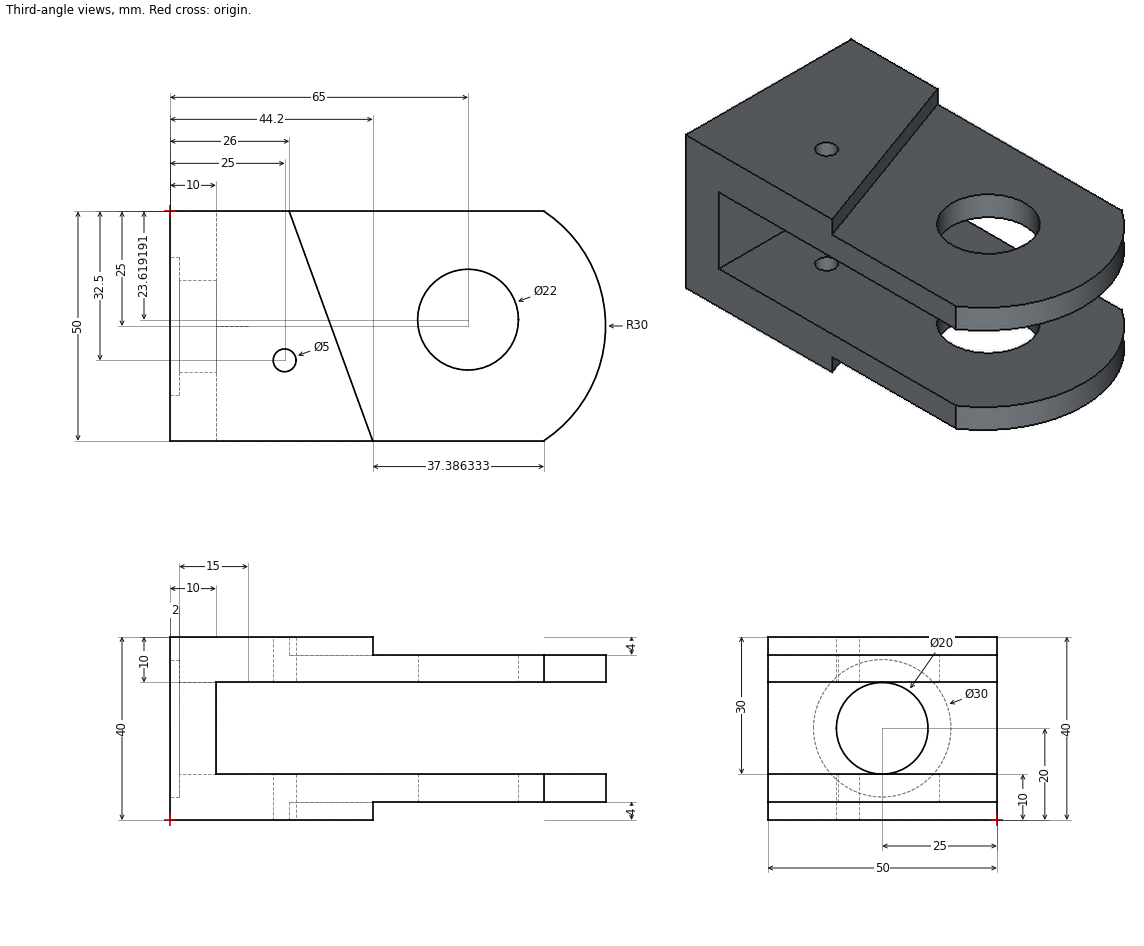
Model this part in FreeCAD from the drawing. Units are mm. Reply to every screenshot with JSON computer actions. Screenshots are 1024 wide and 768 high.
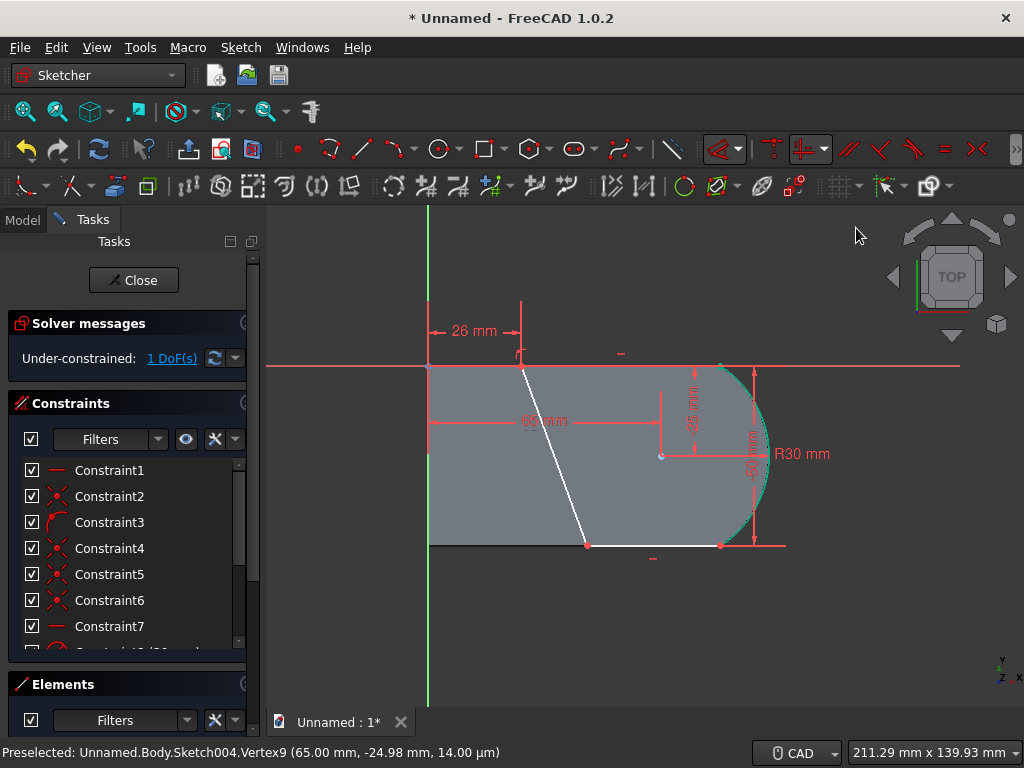
{"action": "left_click", "coordinate": [587, 546]}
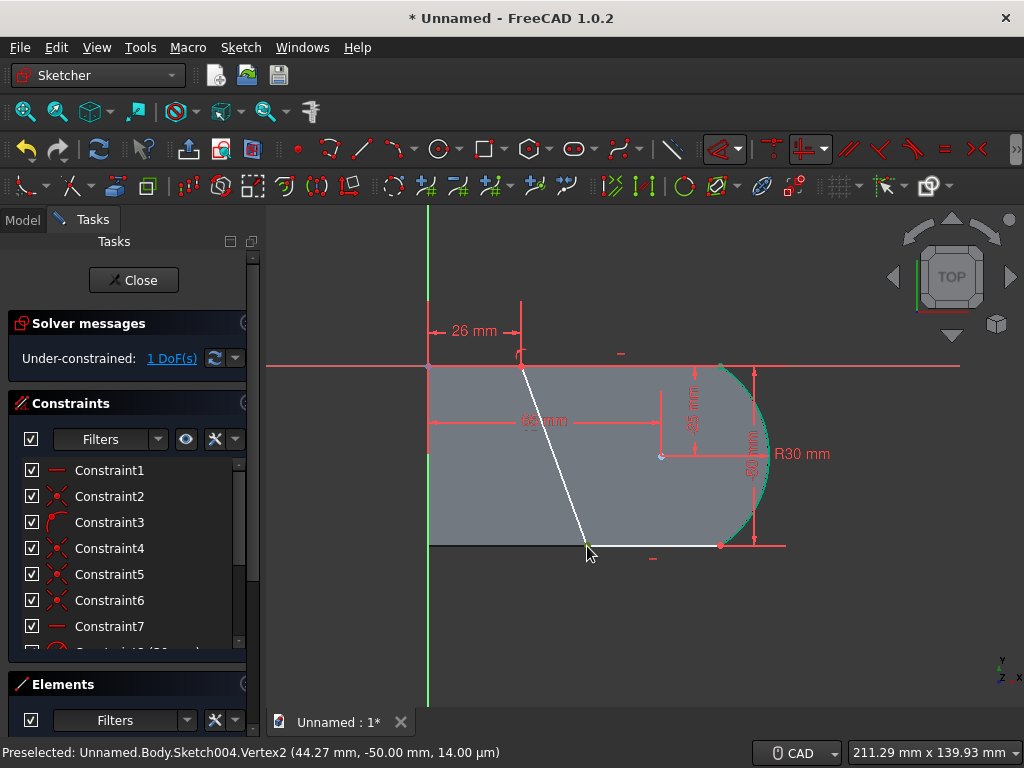
{"action": "key", "text": "l"}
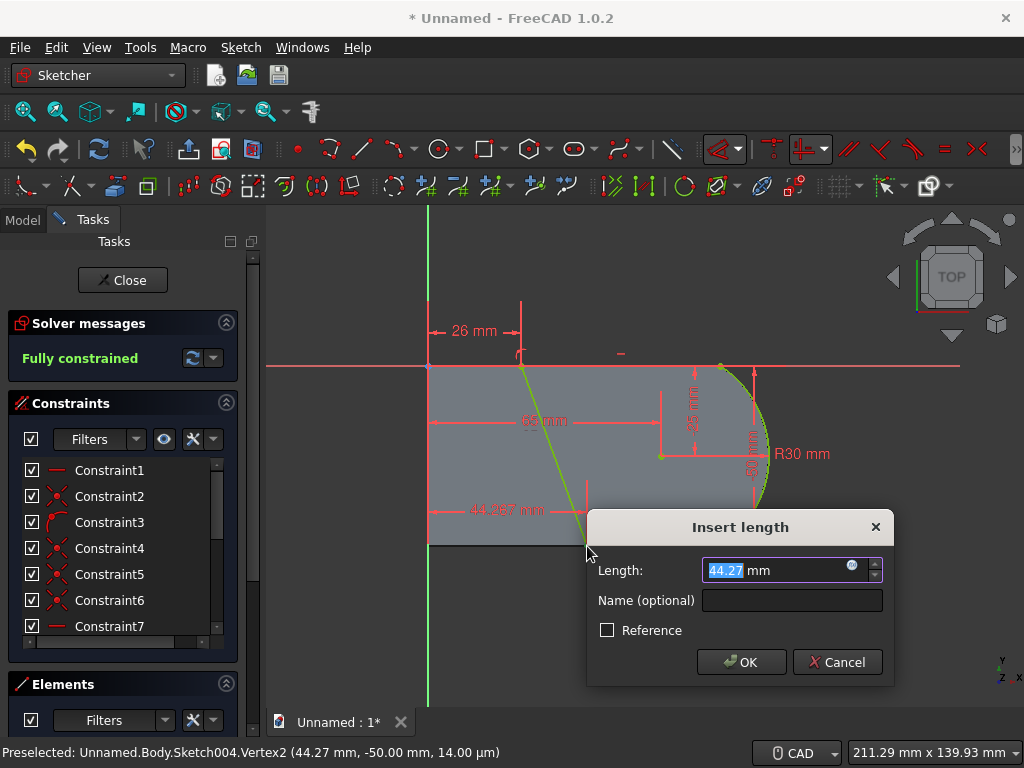
{"action": "type", "text": "44.2"}
{"action": "key", "text": "Return"}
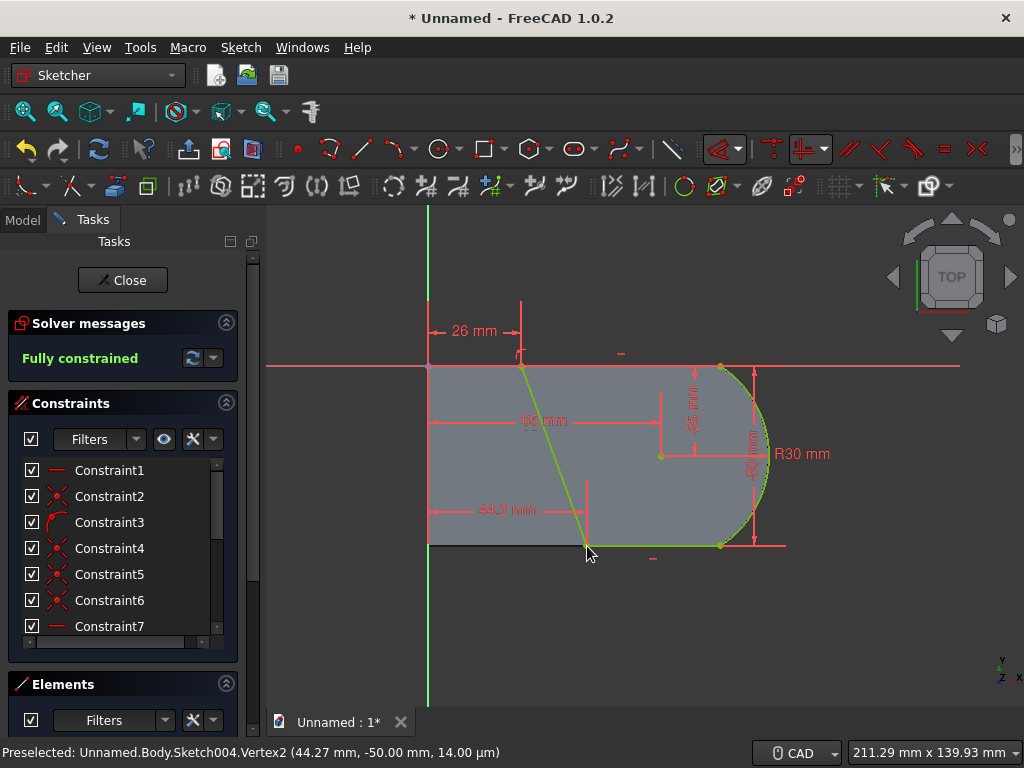
{"action": "left_click", "coordinate": [123, 280]}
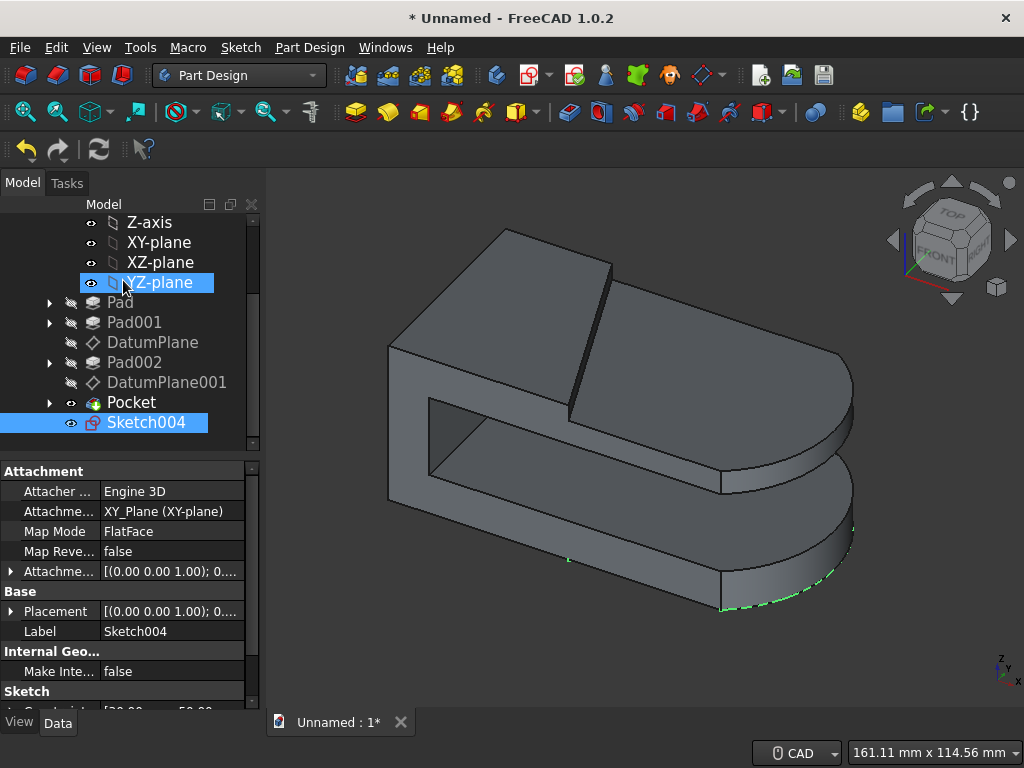
{"action": "left_click", "coordinate": [570, 112]}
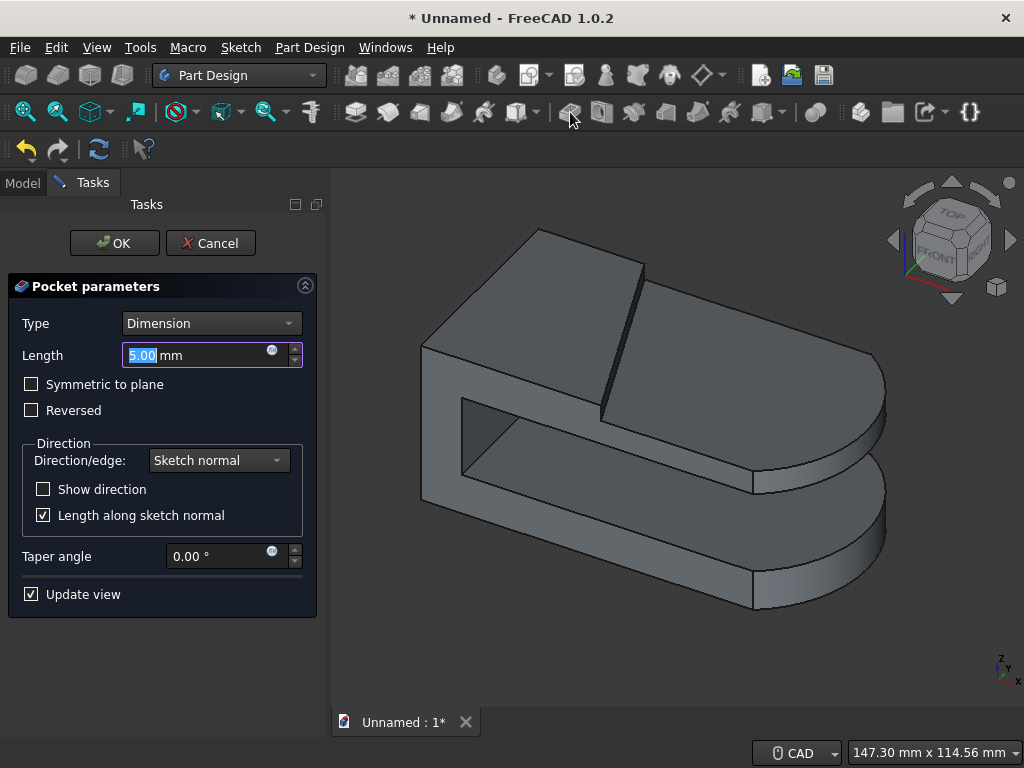
{"action": "type", "text": "4"}
{"action": "key", "text": "Tab"}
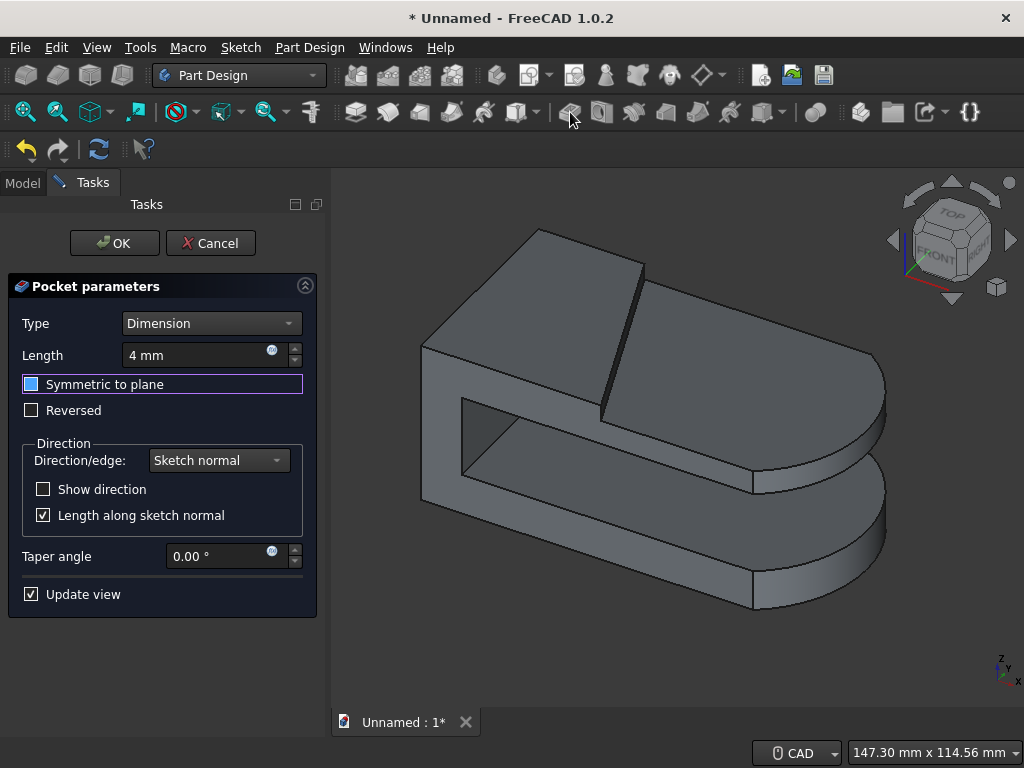
{"action": "left_click", "coordinate": [30, 410]}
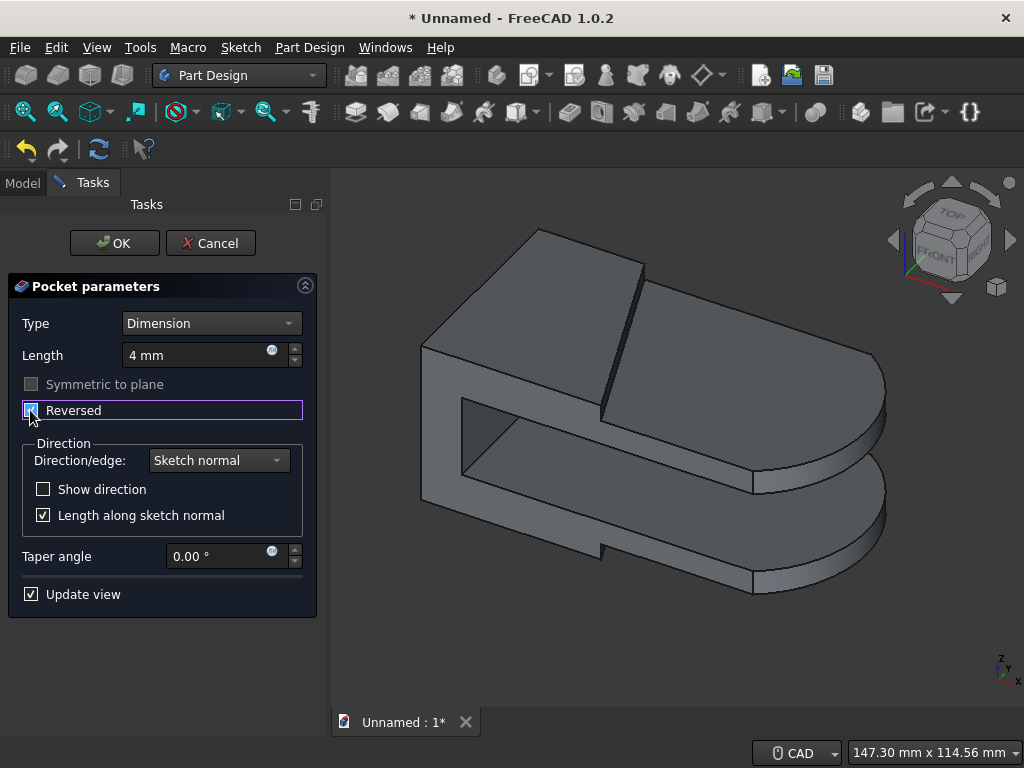
{"action": "left_click", "coordinate": [115, 243]}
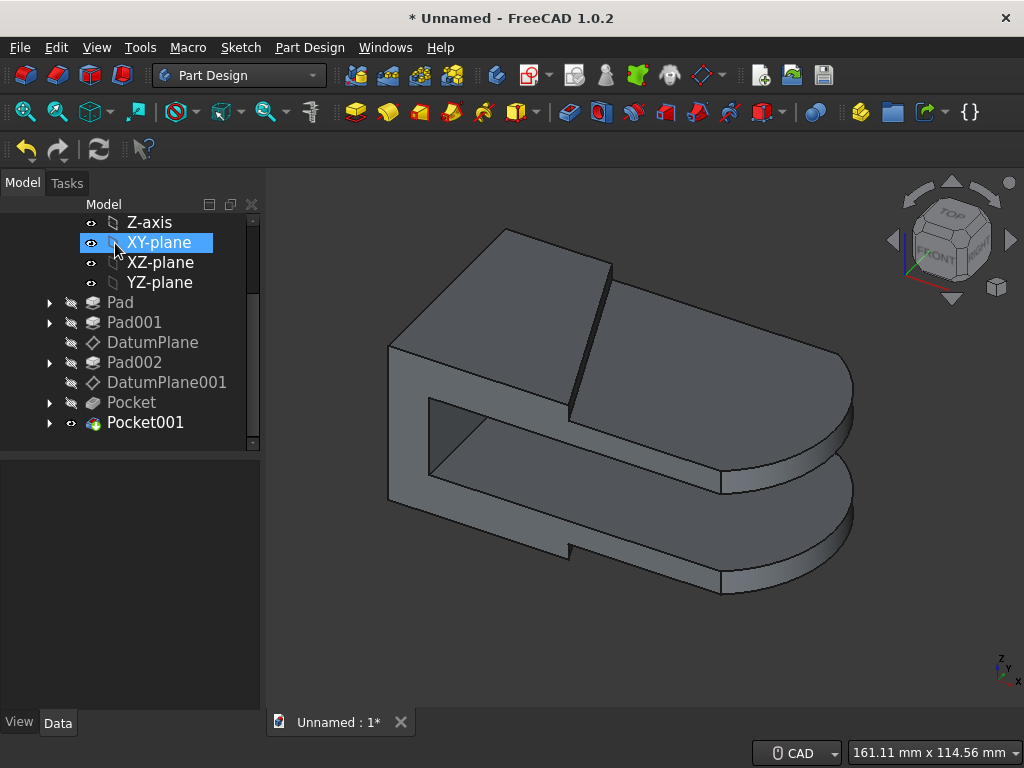
{"action": "left_click", "coordinate": [734, 397]}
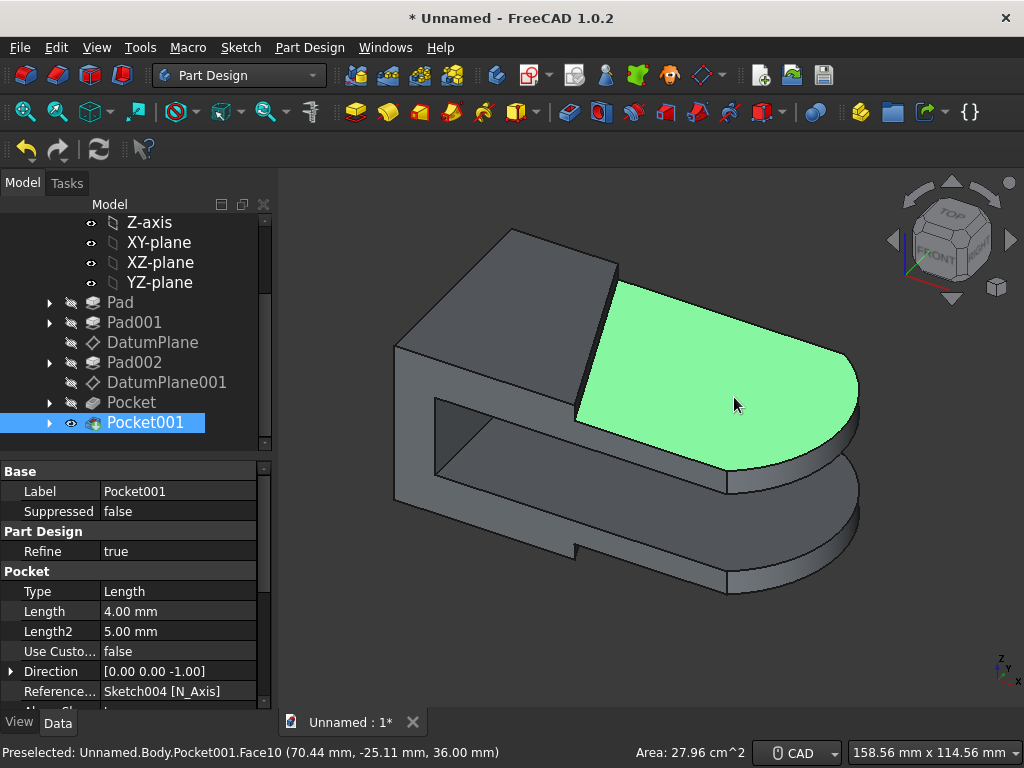
{"action": "left_click", "coordinate": [530, 76]}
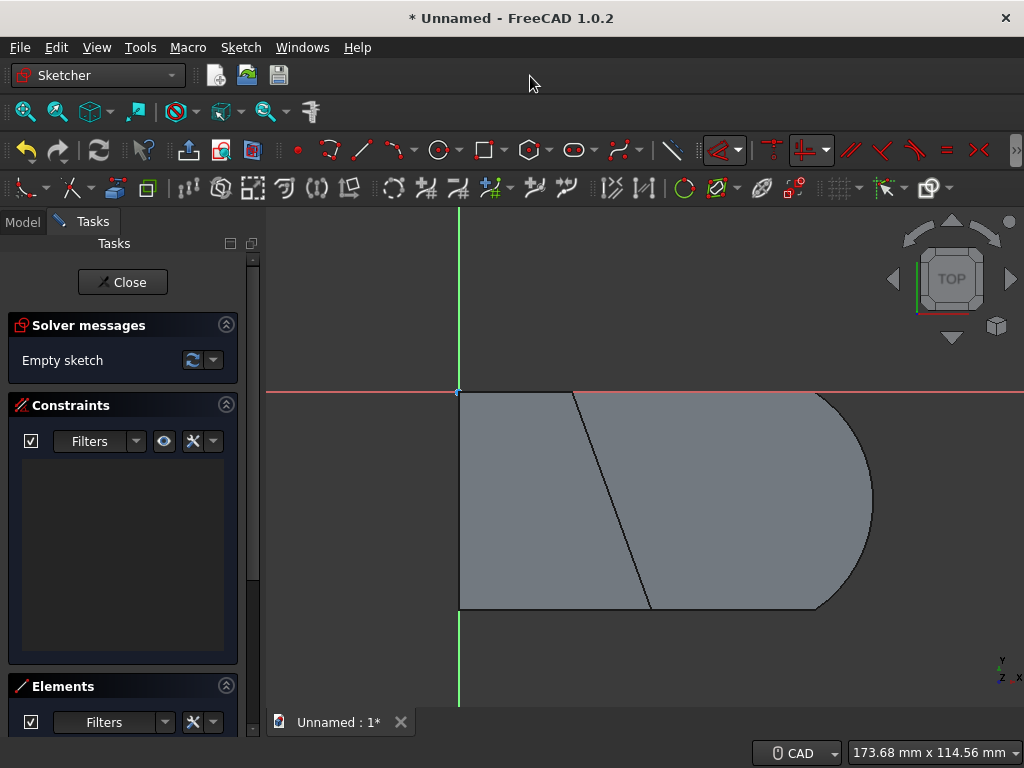
{"action": "left_click", "coordinate": [254, 150]}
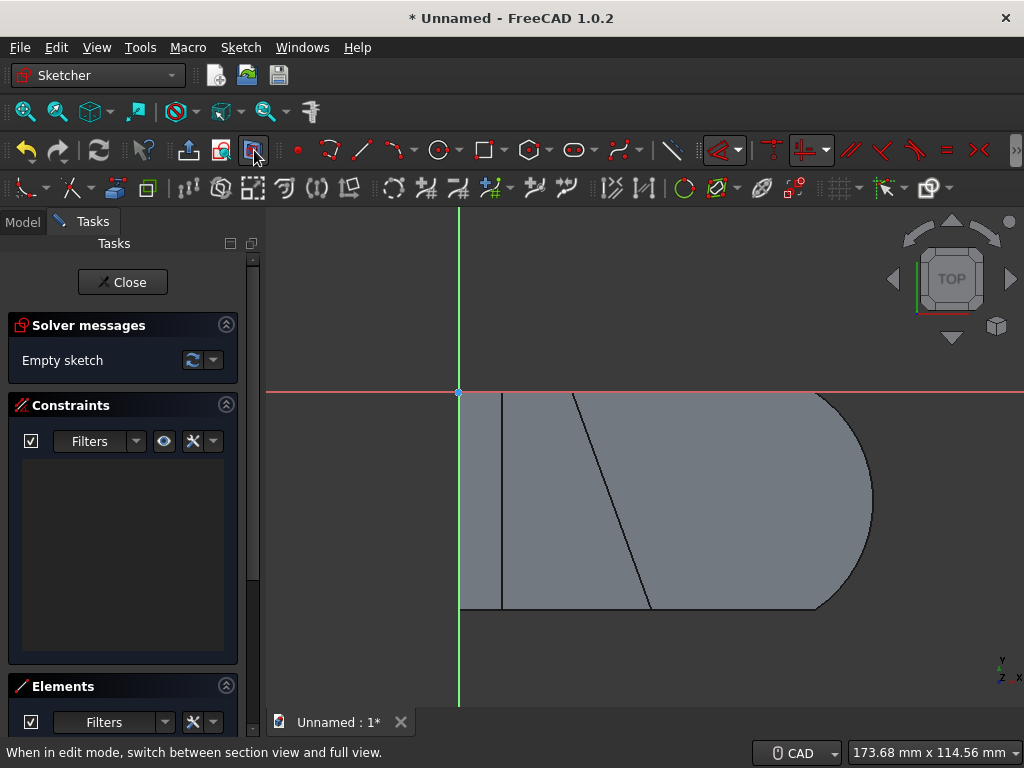
{"action": "scroll", "coordinate": [814, 512], "scroll_direction": "up", "scroll_amount": 6}